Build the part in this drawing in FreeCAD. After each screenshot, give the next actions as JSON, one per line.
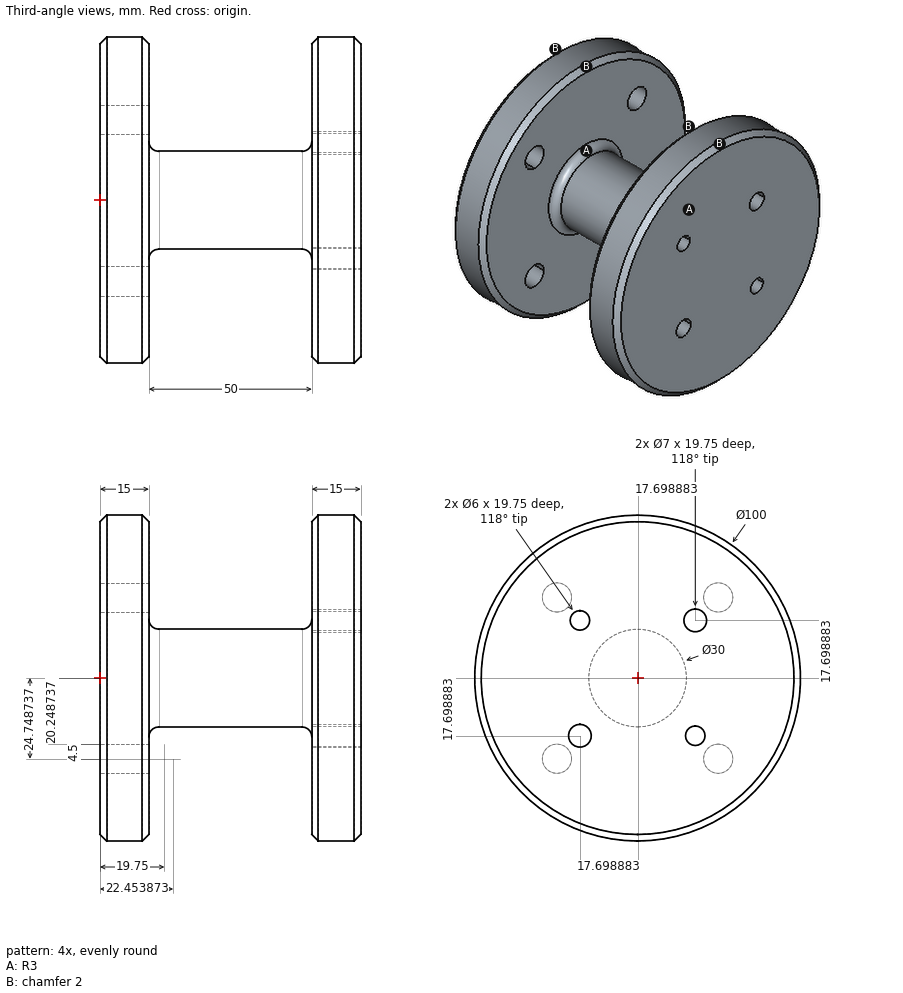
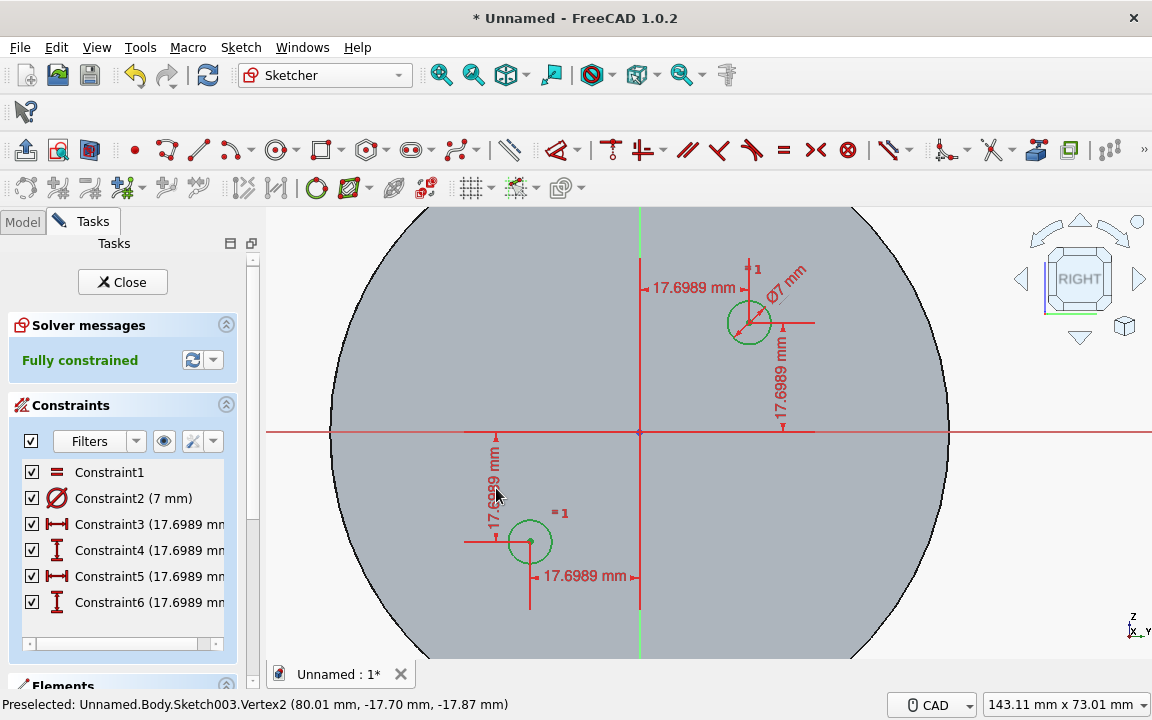
{"action": "left_click", "coordinate": [123, 282]}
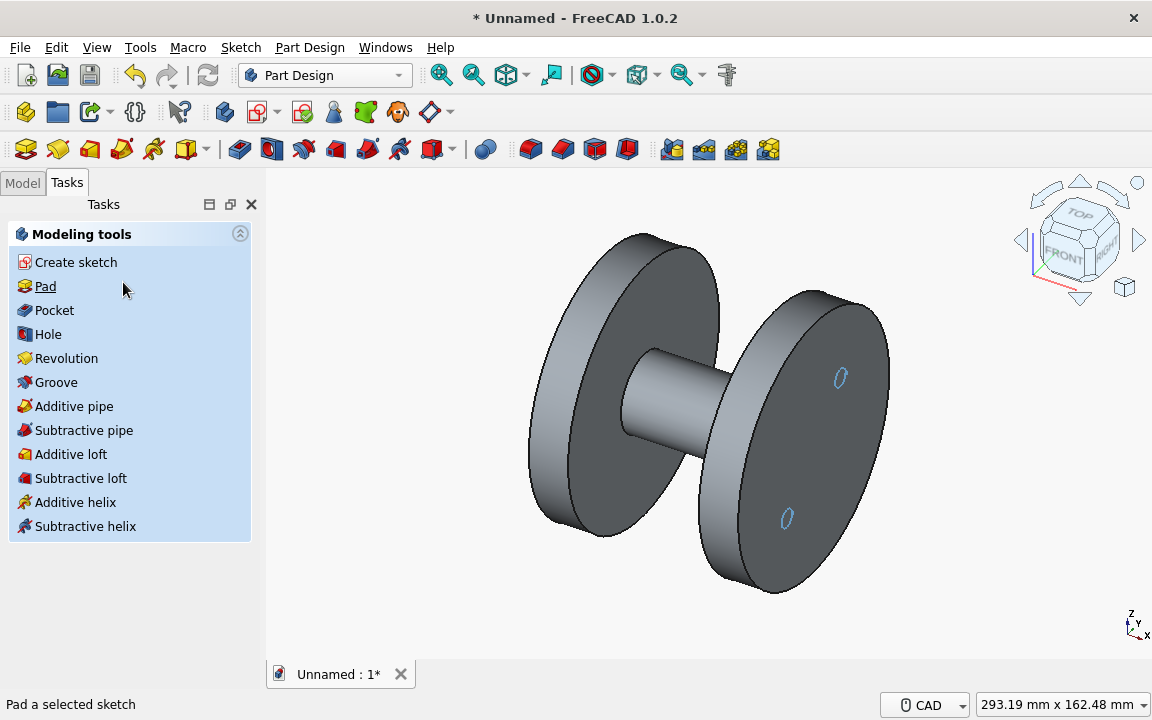
{"action": "left_click", "coordinate": [272, 150]}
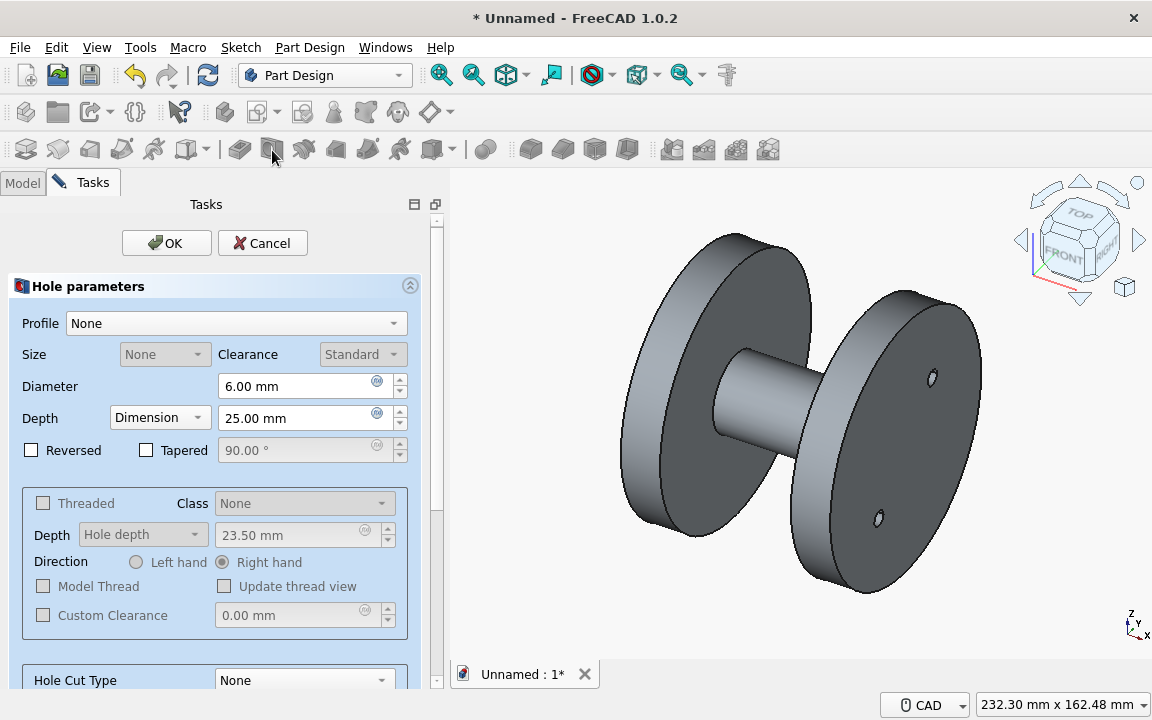
{"action": "triple_click", "coordinate": [305, 386]}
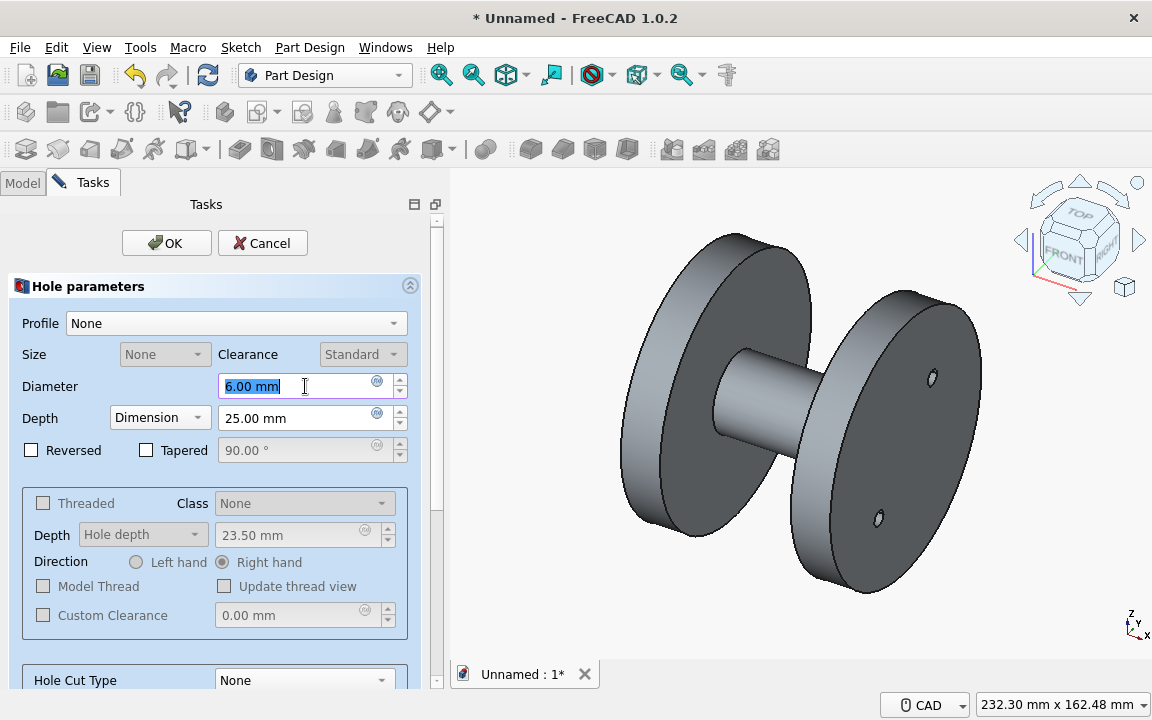
{"action": "type", "text": "7"}
{"action": "key", "text": "Tab"}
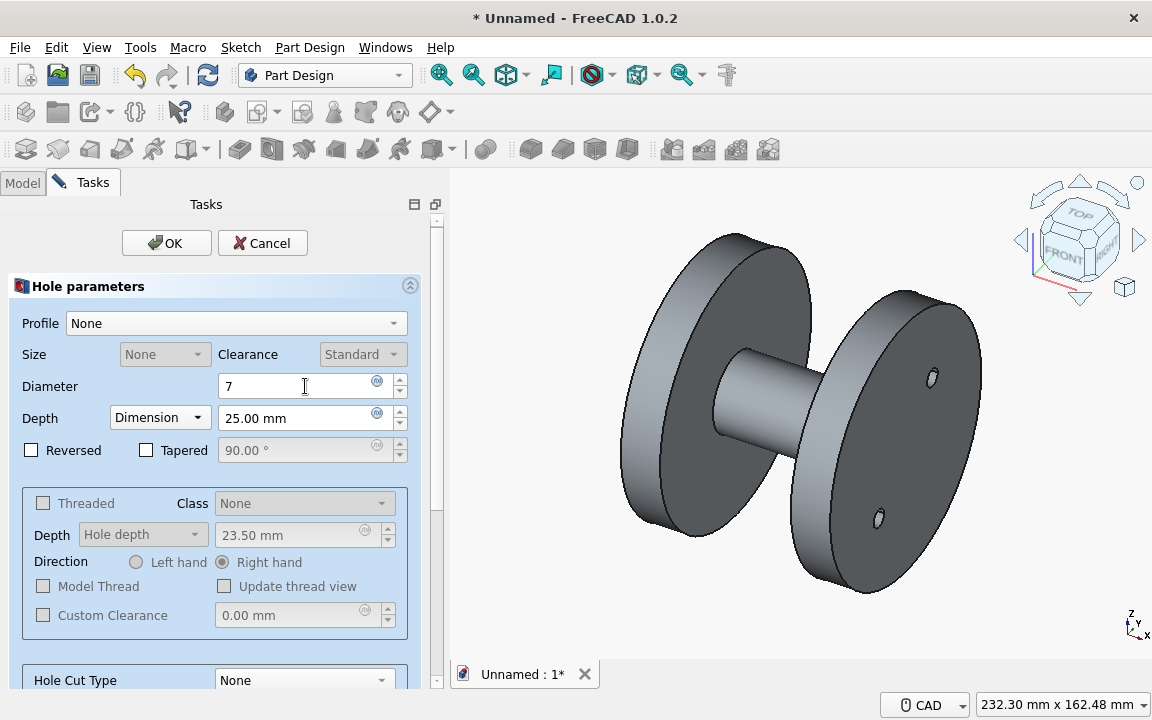
{"action": "triple_click", "coordinate": [305, 418]}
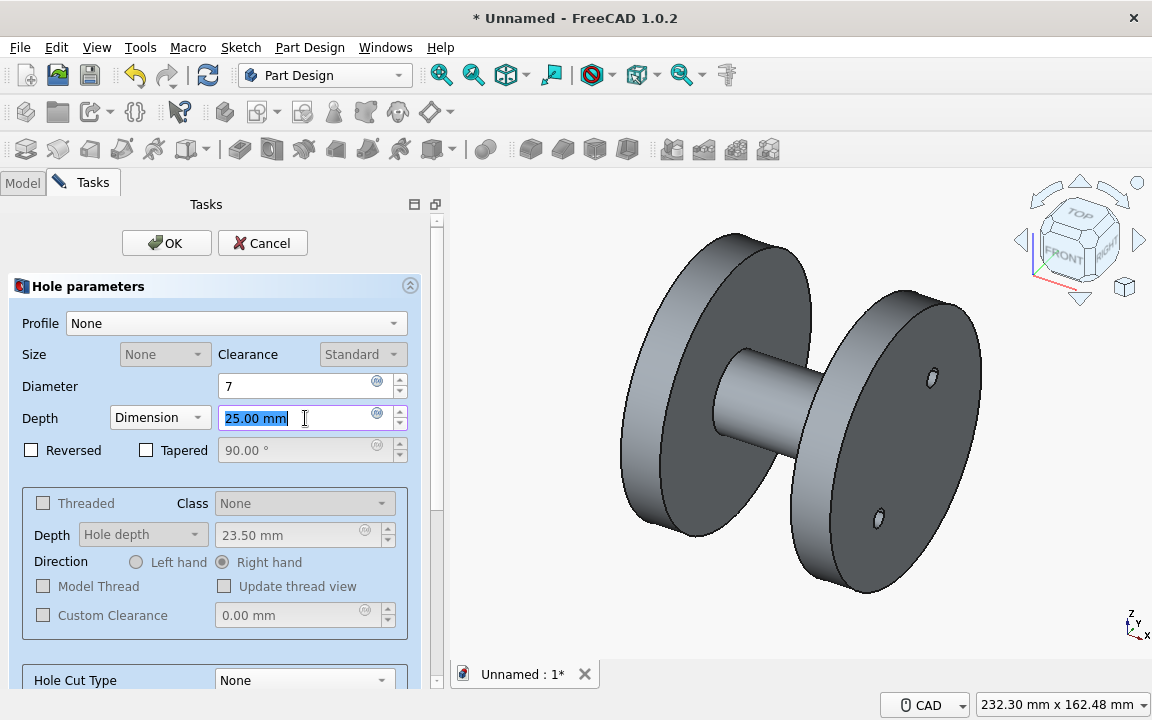
{"action": "type", "text": "19.75"}
{"action": "key", "text": "Tab"}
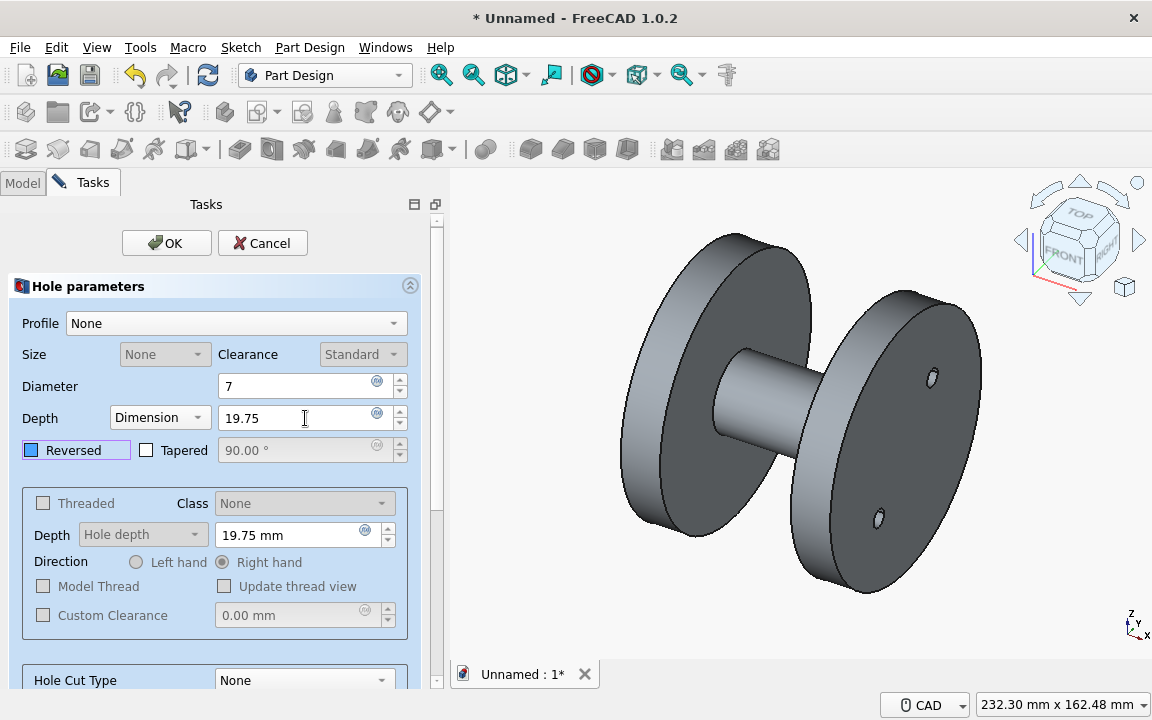
{"action": "left_click", "coordinate": [167, 243]}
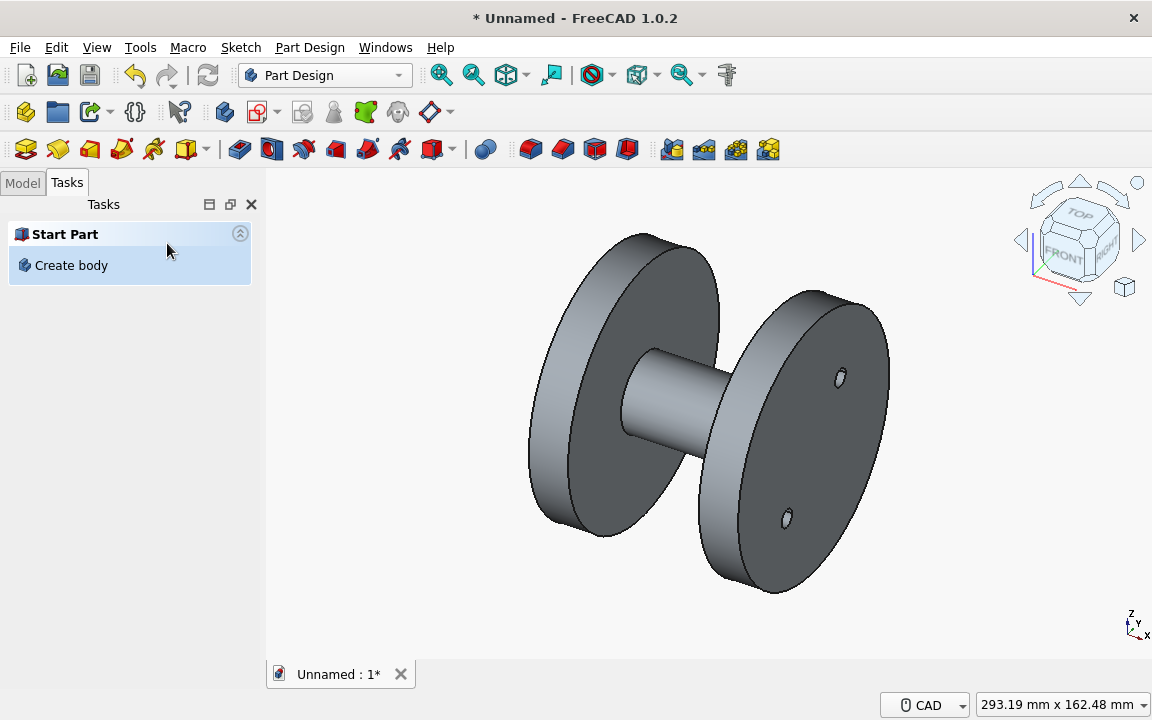
{"action": "left_click", "coordinate": [792, 433]}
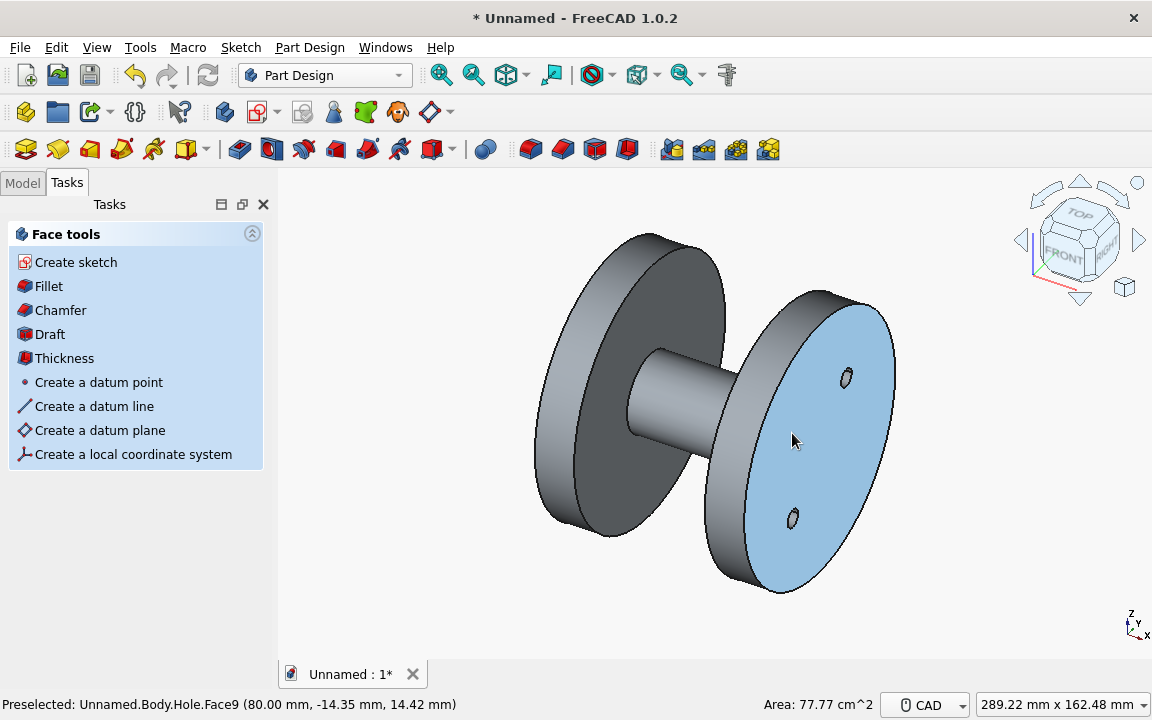
{"action": "left_click", "coordinate": [258, 112]}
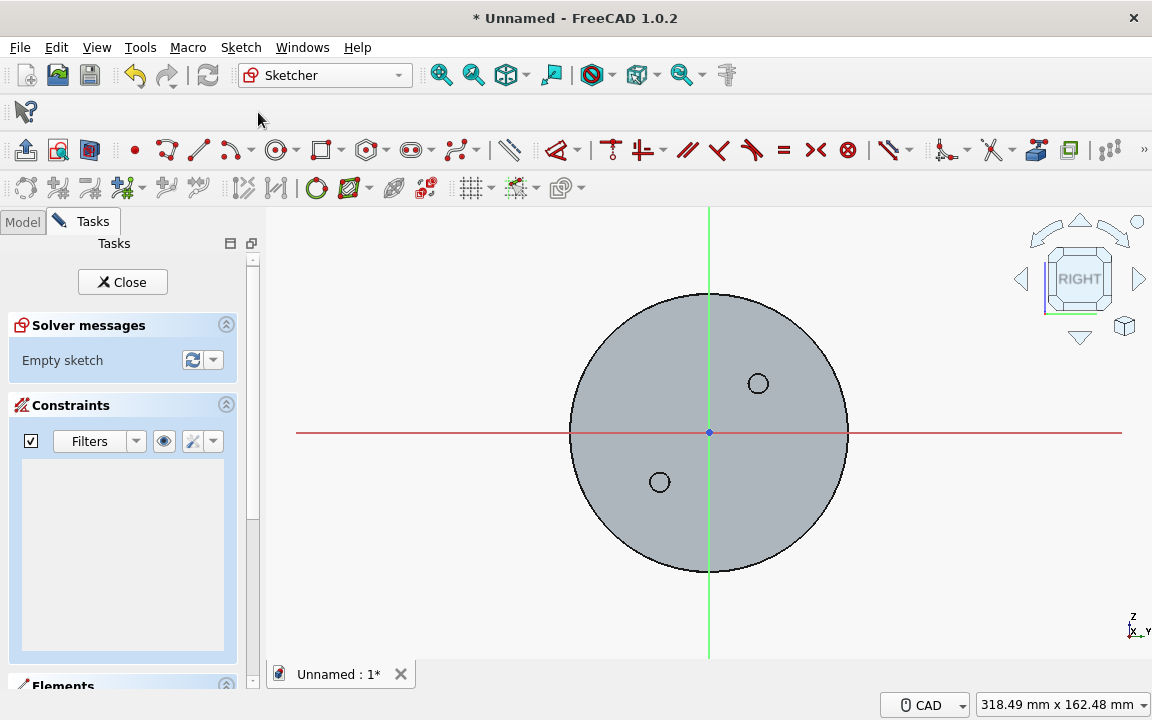
{"action": "scroll", "coordinate": [765, 433], "scroll_direction": "up", "scroll_amount": 4}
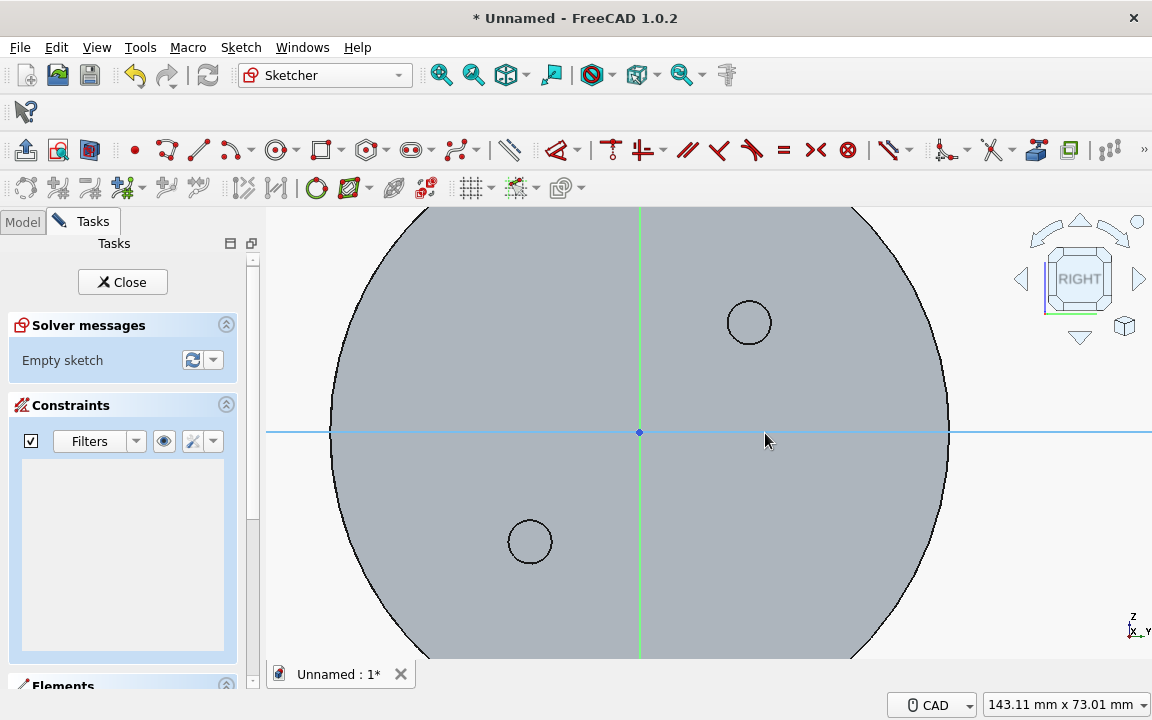
{"action": "left_click", "coordinate": [276, 150]}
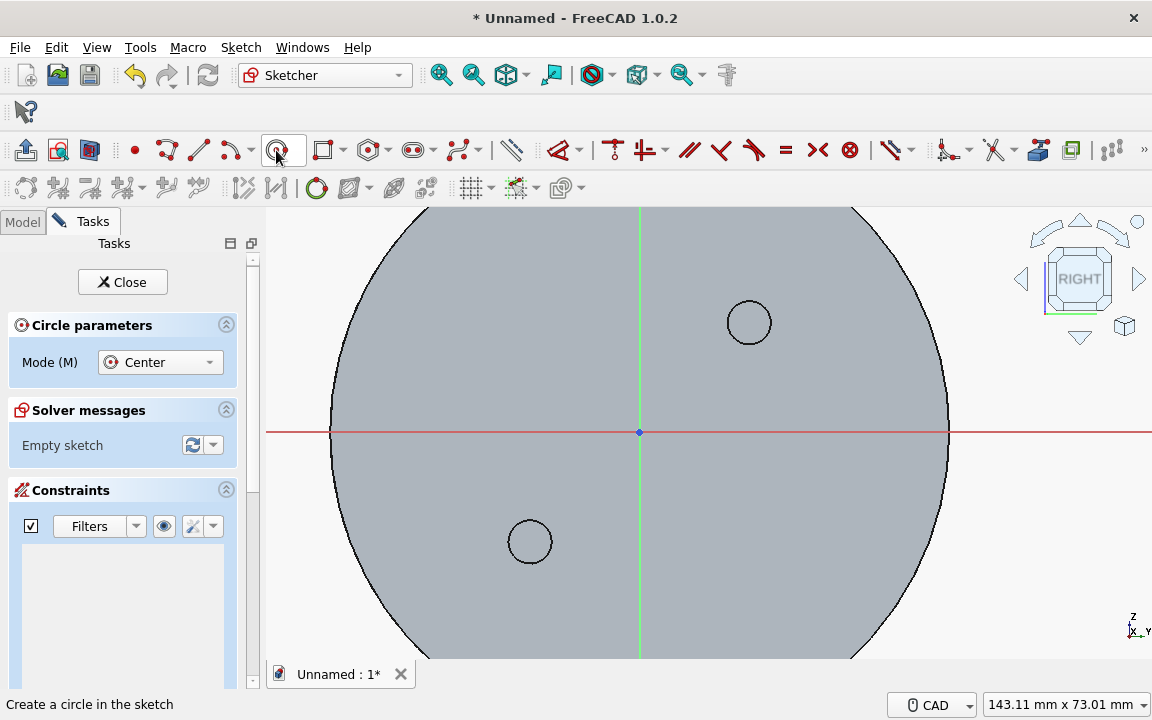
{"action": "left_click", "coordinate": [530, 323]}
{"action": "left_click", "coordinate": [543, 310]}